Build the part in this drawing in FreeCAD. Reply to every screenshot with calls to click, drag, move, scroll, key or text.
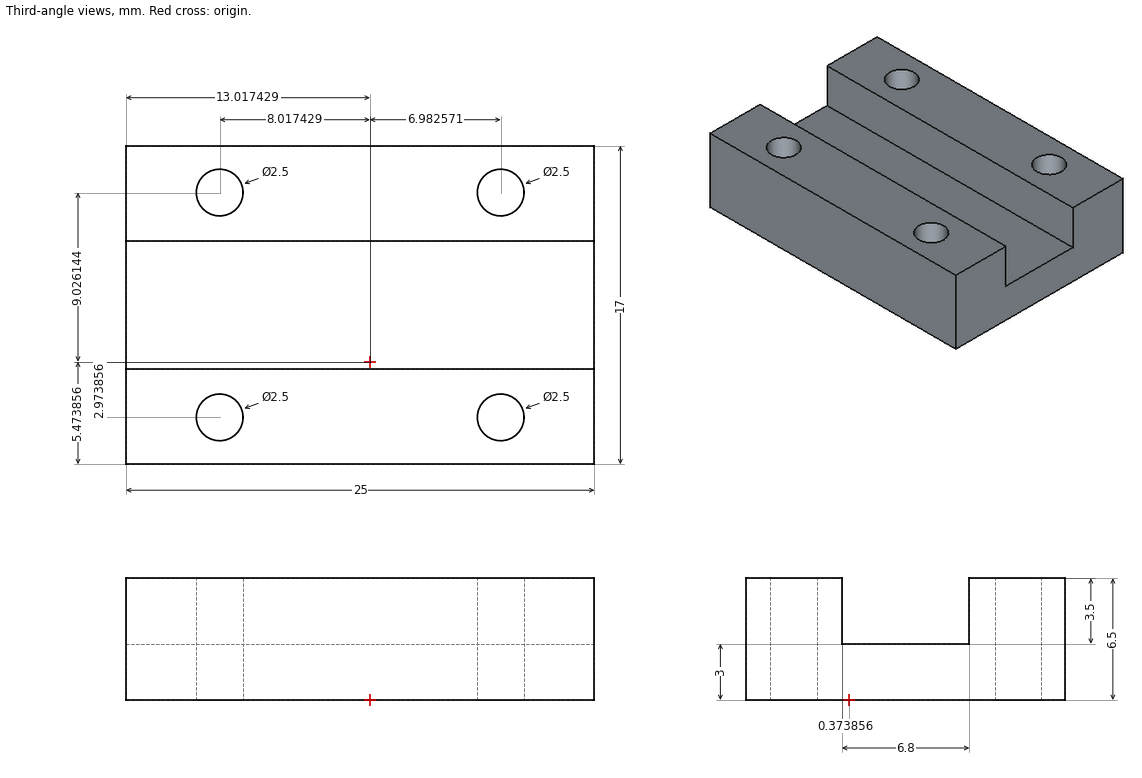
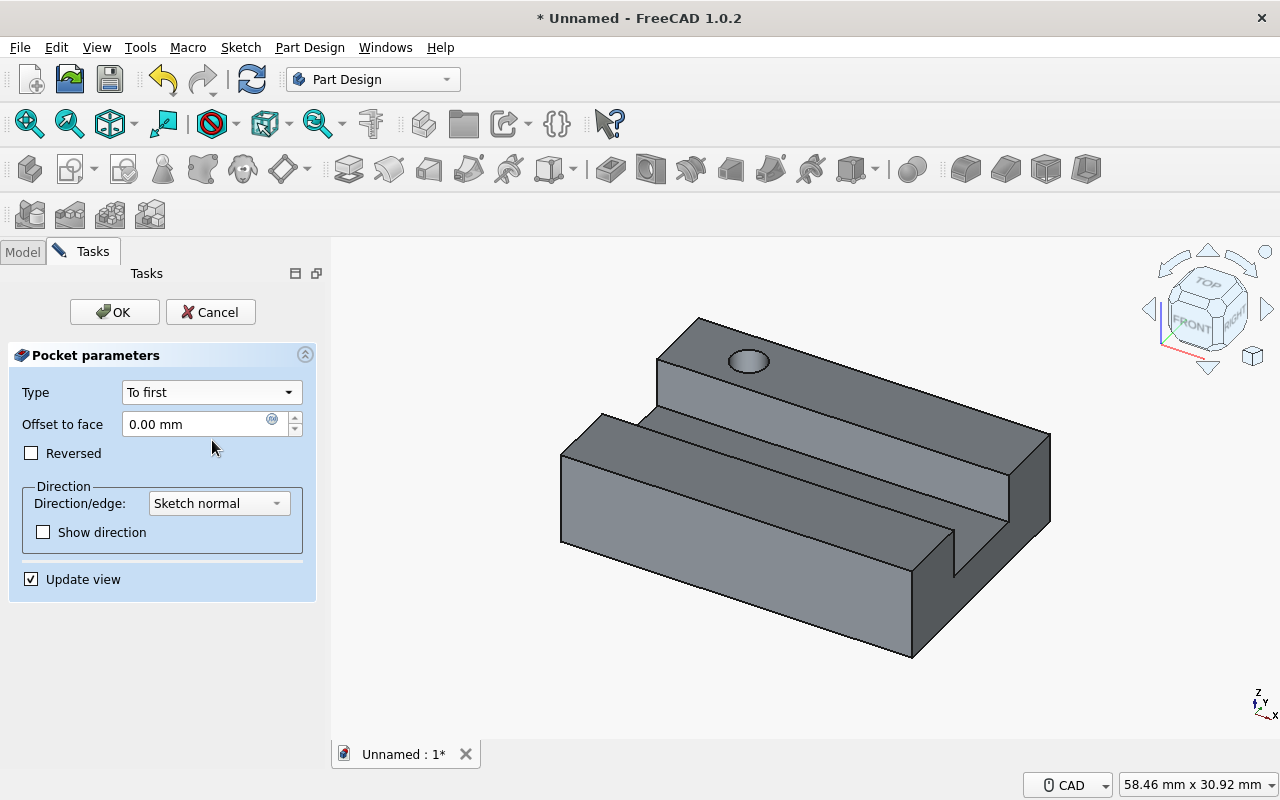
click(115, 312)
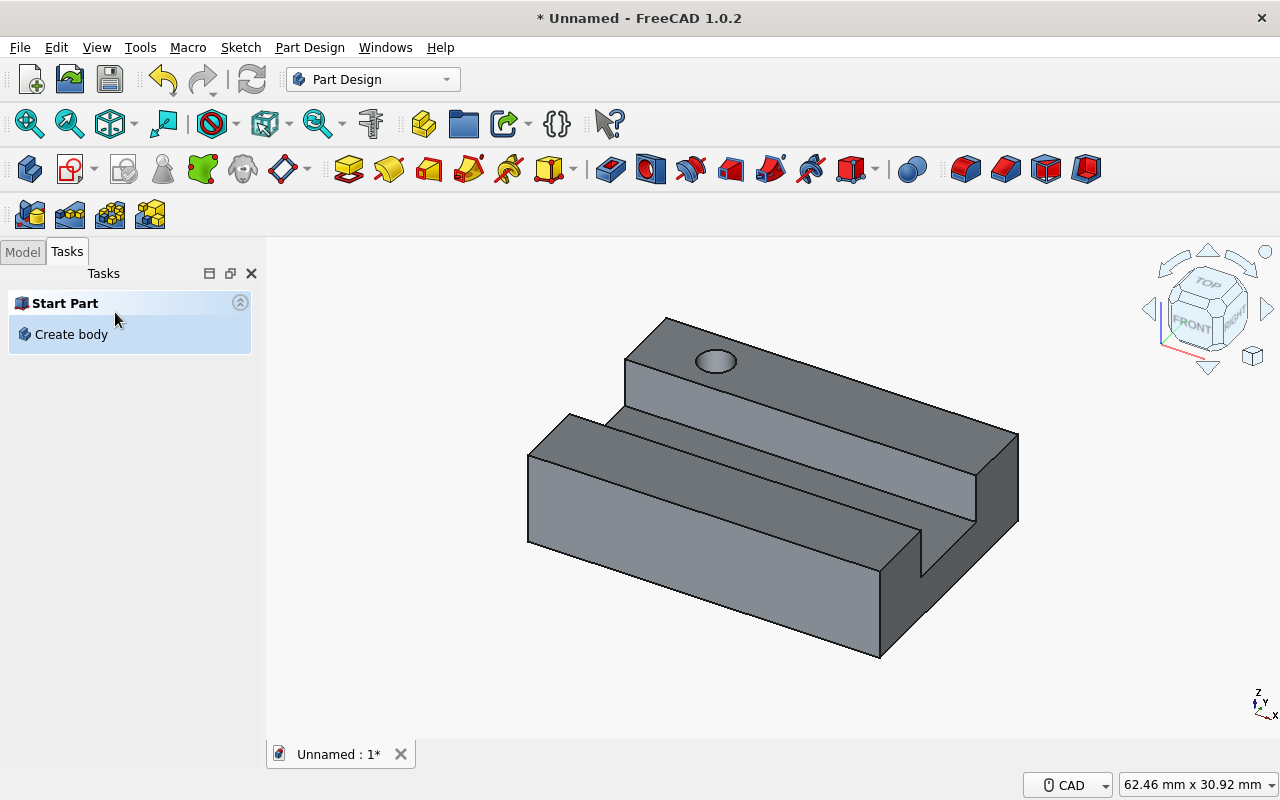
click(825, 525)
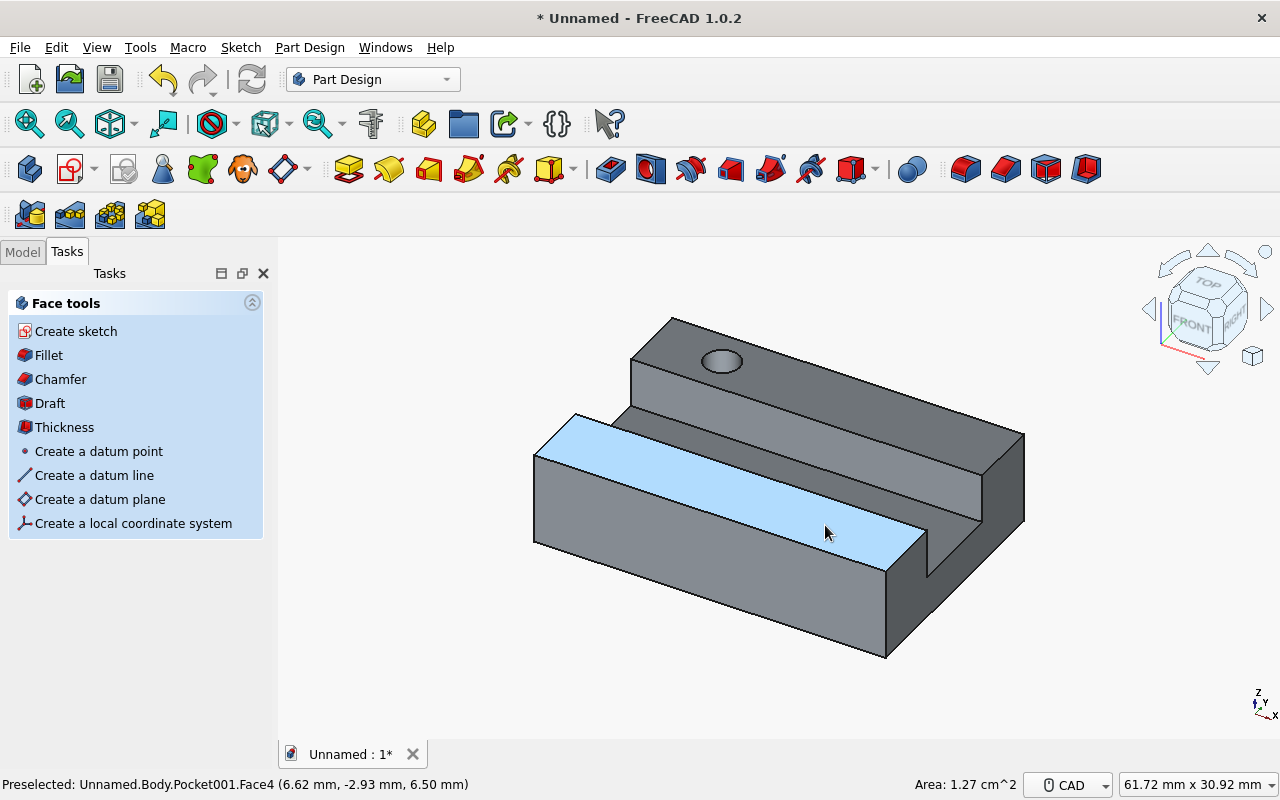
click(70, 170)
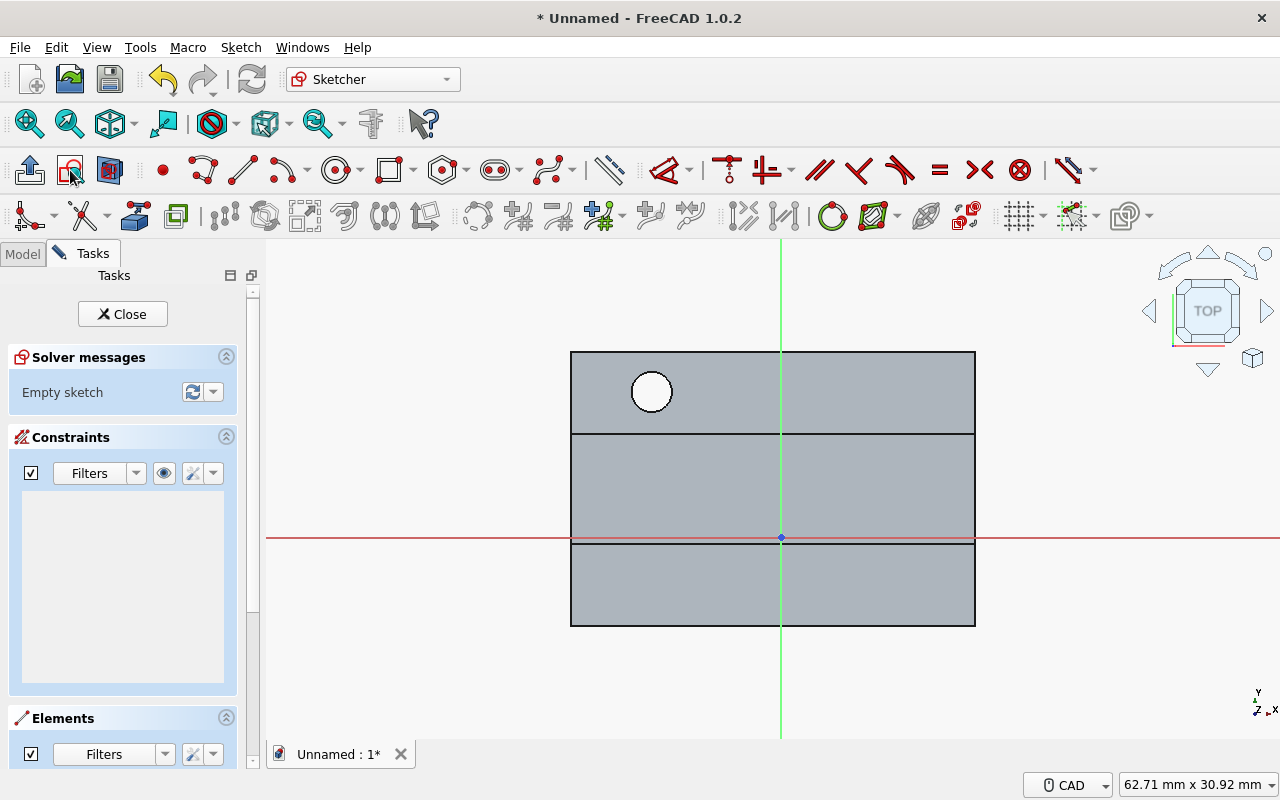
scroll(924, 377, up, 10)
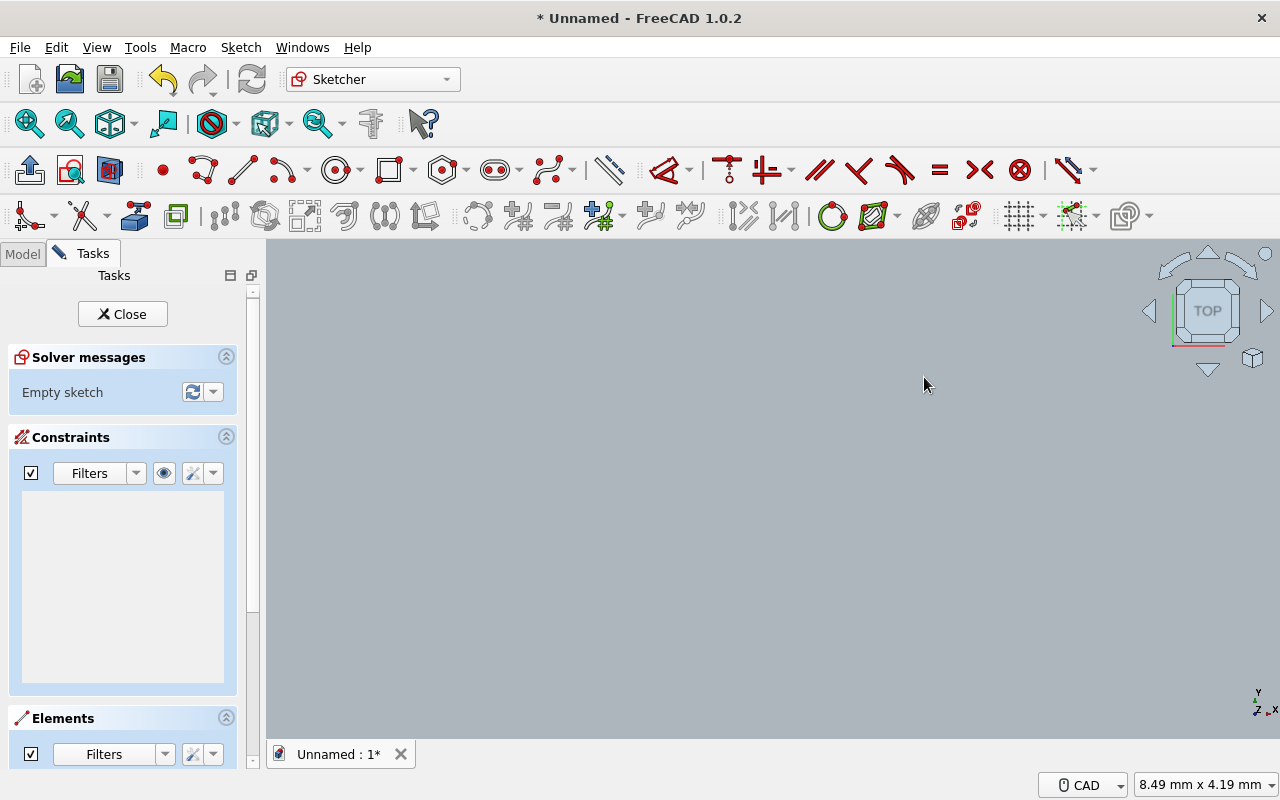
key(g)
key(c)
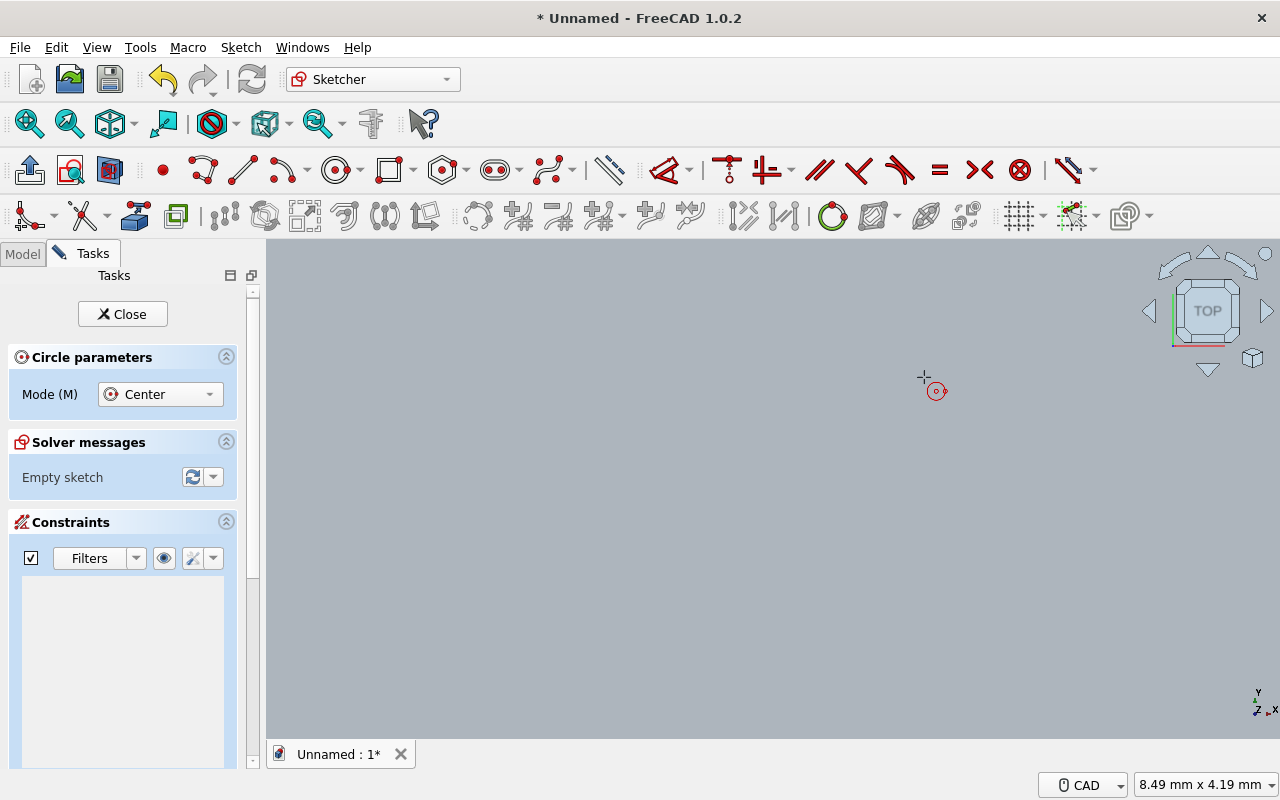
click(700, 486)
move(806, 380)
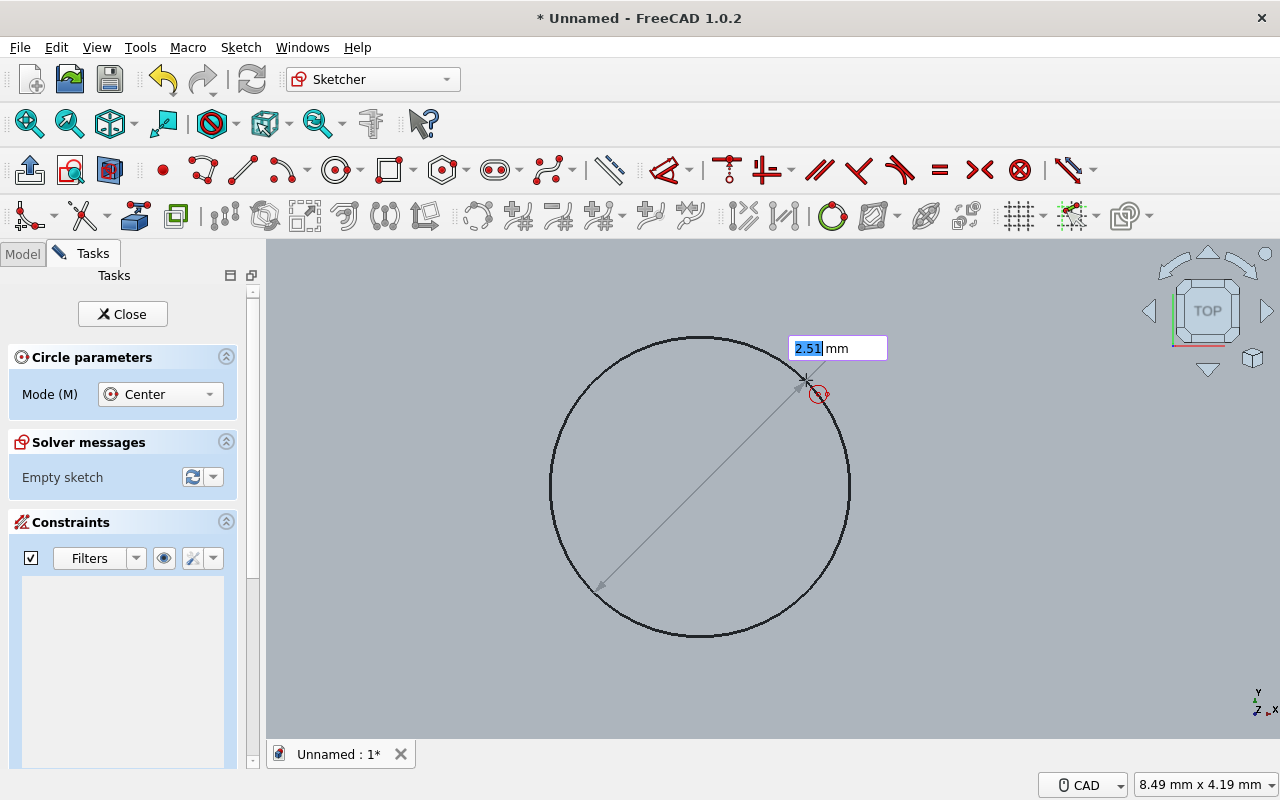
text(2.5)
key(Return)
key(Escape)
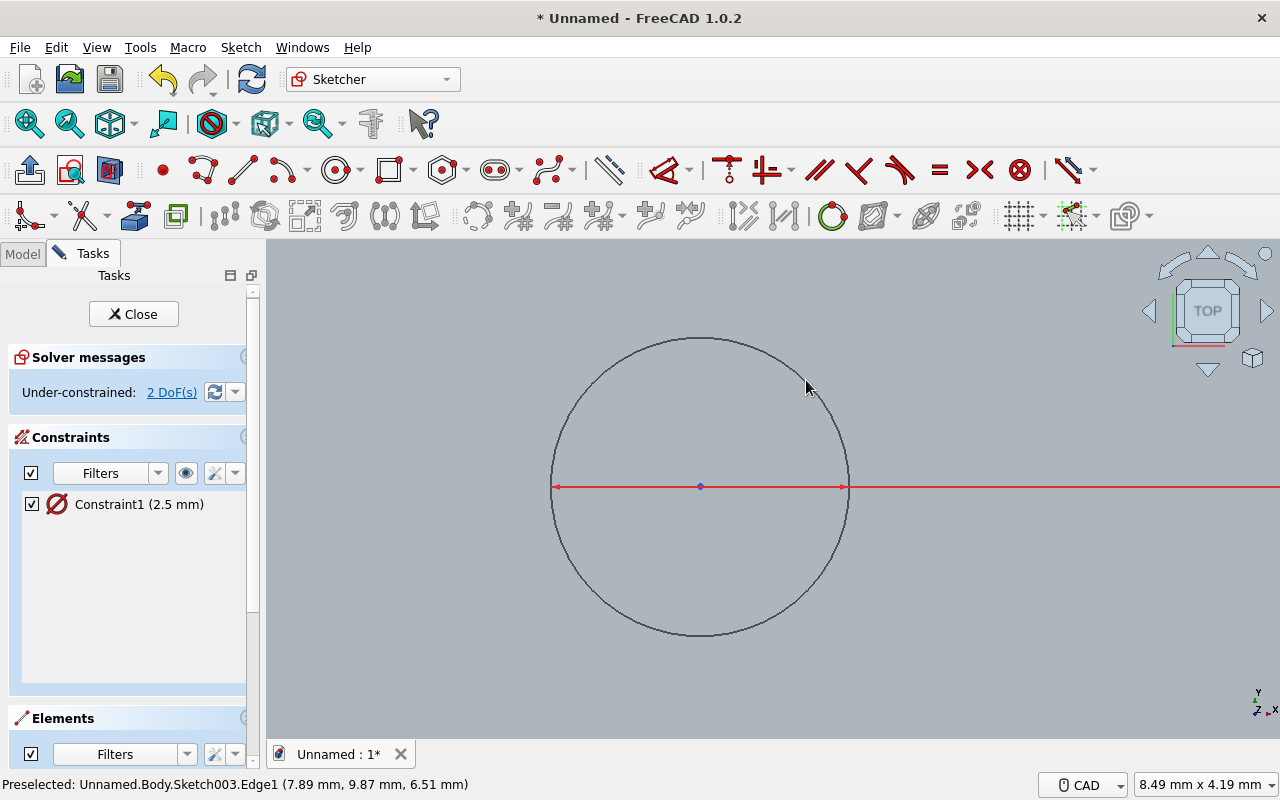
click(664, 170)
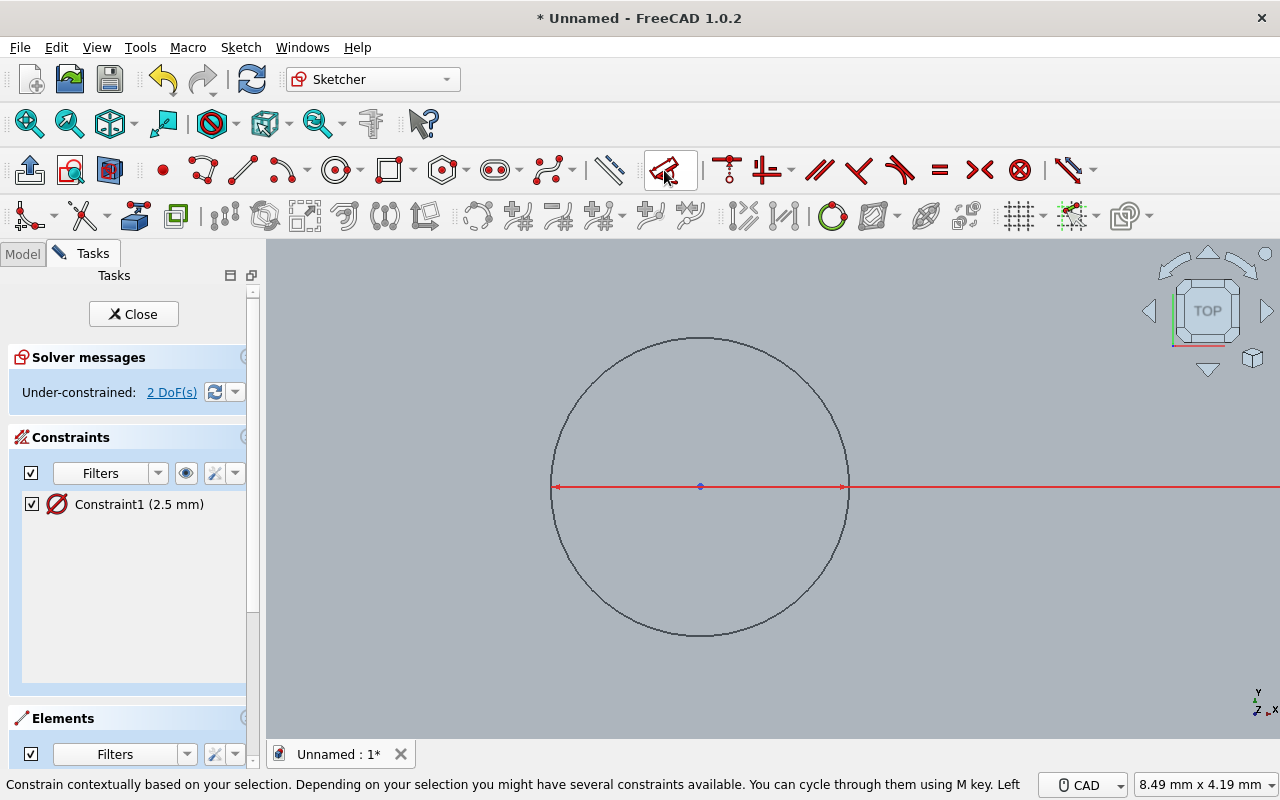
click(700, 487)
click(497, 453)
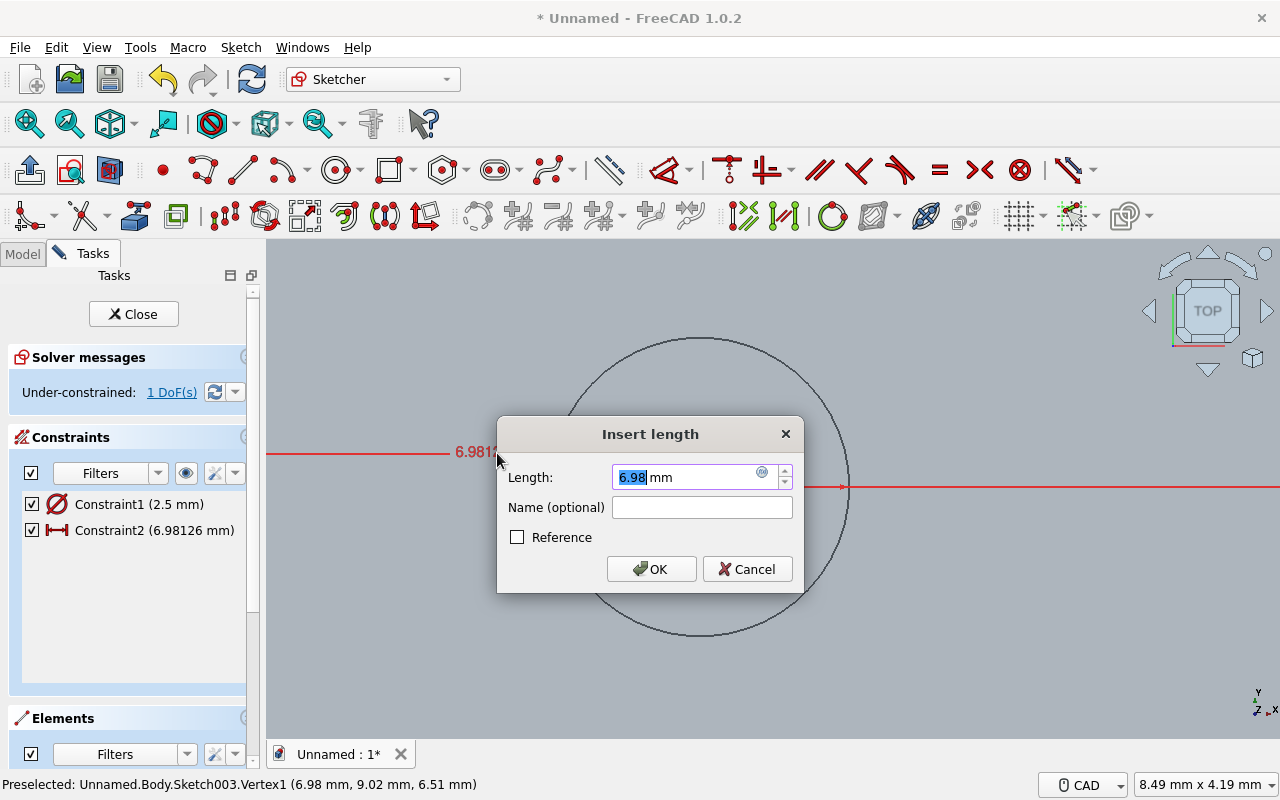
text(6.982571)
key(Return)